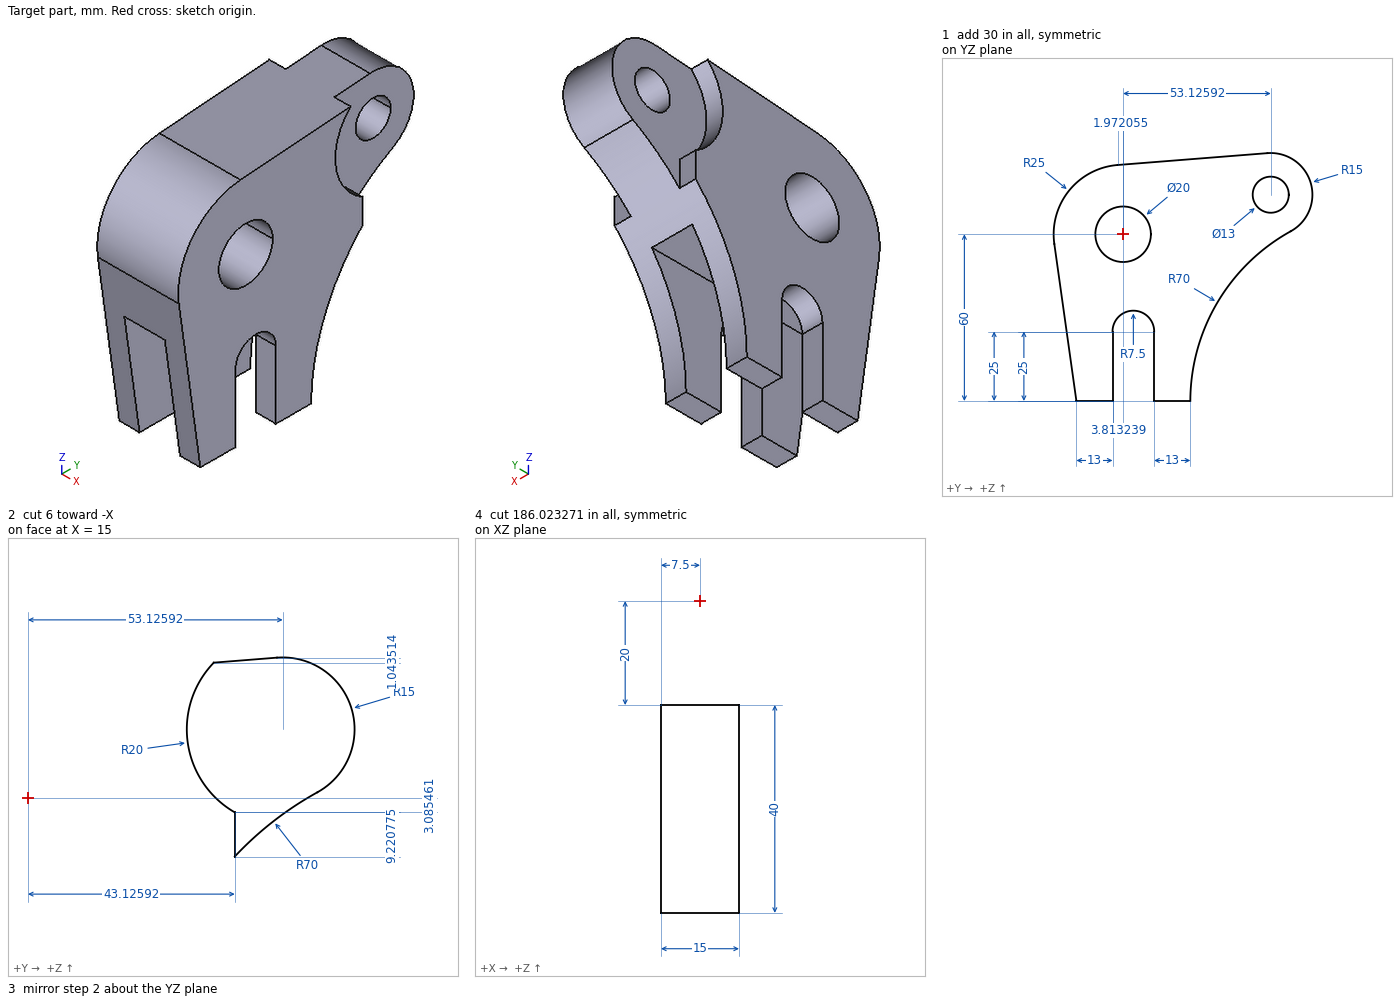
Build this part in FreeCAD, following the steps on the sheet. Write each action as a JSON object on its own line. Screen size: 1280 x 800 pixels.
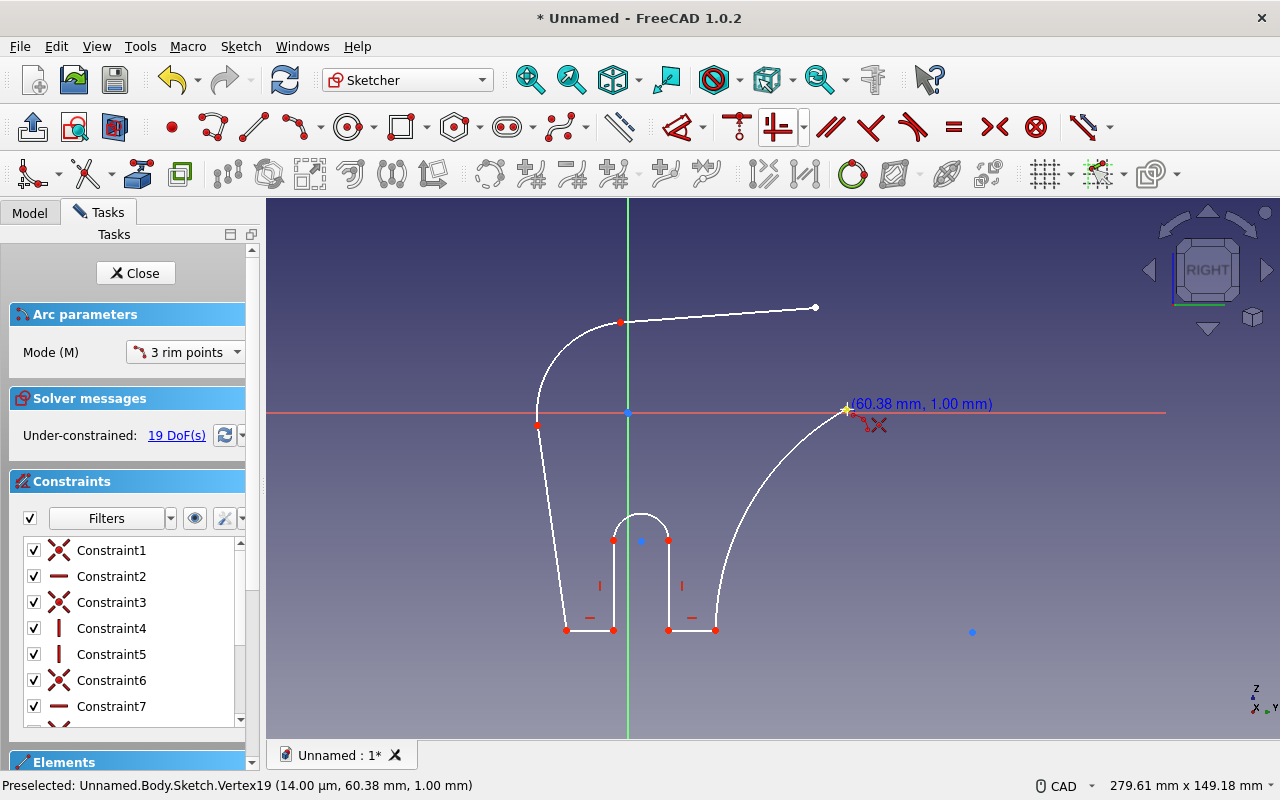
{"action": "left_click", "coordinate": [816, 308]}
{"action": "left_click", "coordinate": [872, 345]}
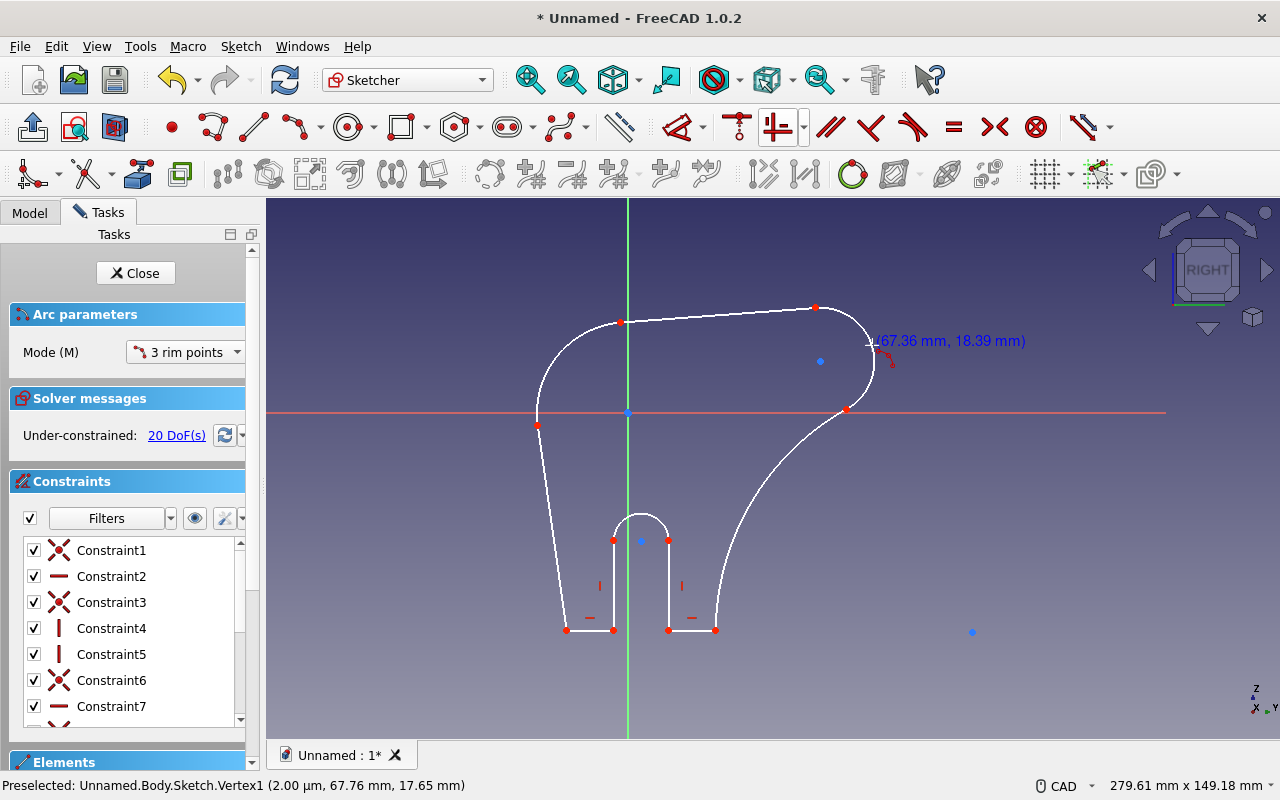
{"action": "left_click", "coordinate": [348, 128]}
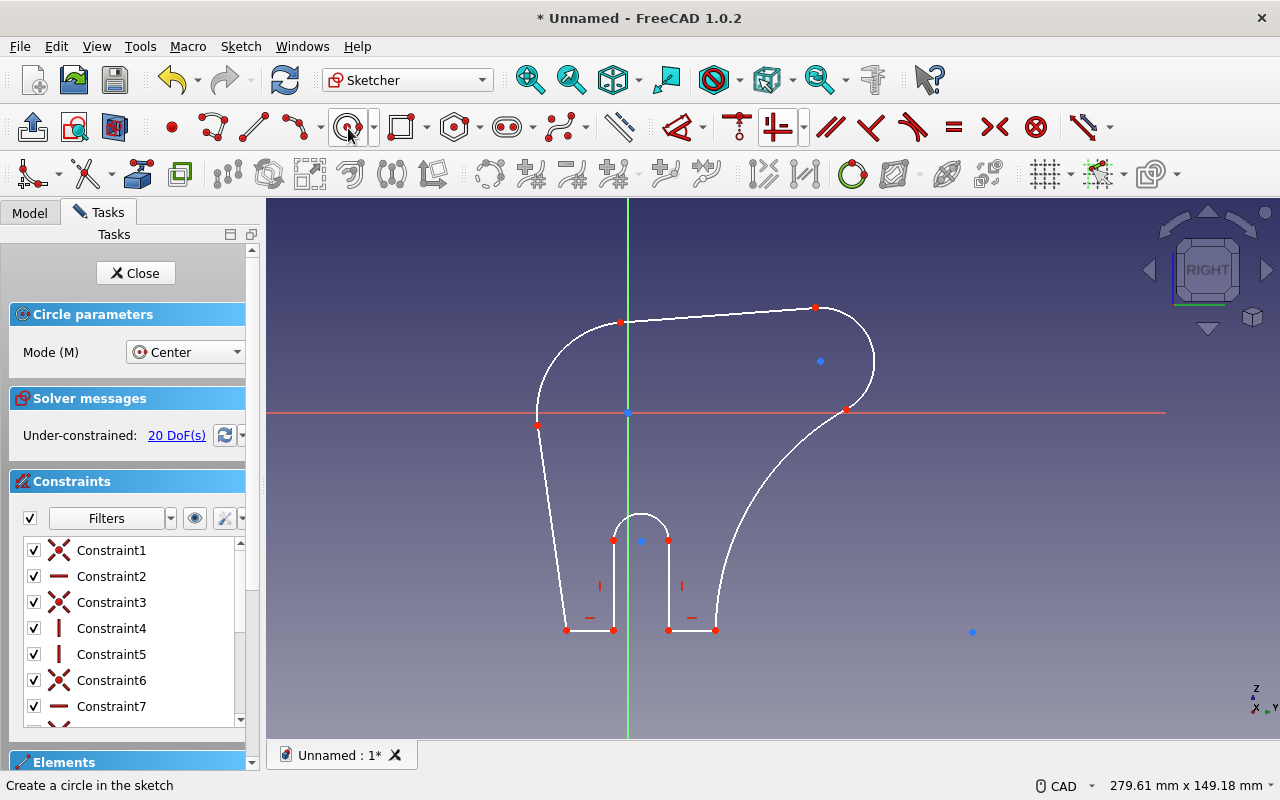
{"action": "left_click", "coordinate": [628, 413]}
{"action": "mouse_move", "coordinate": [653, 387]}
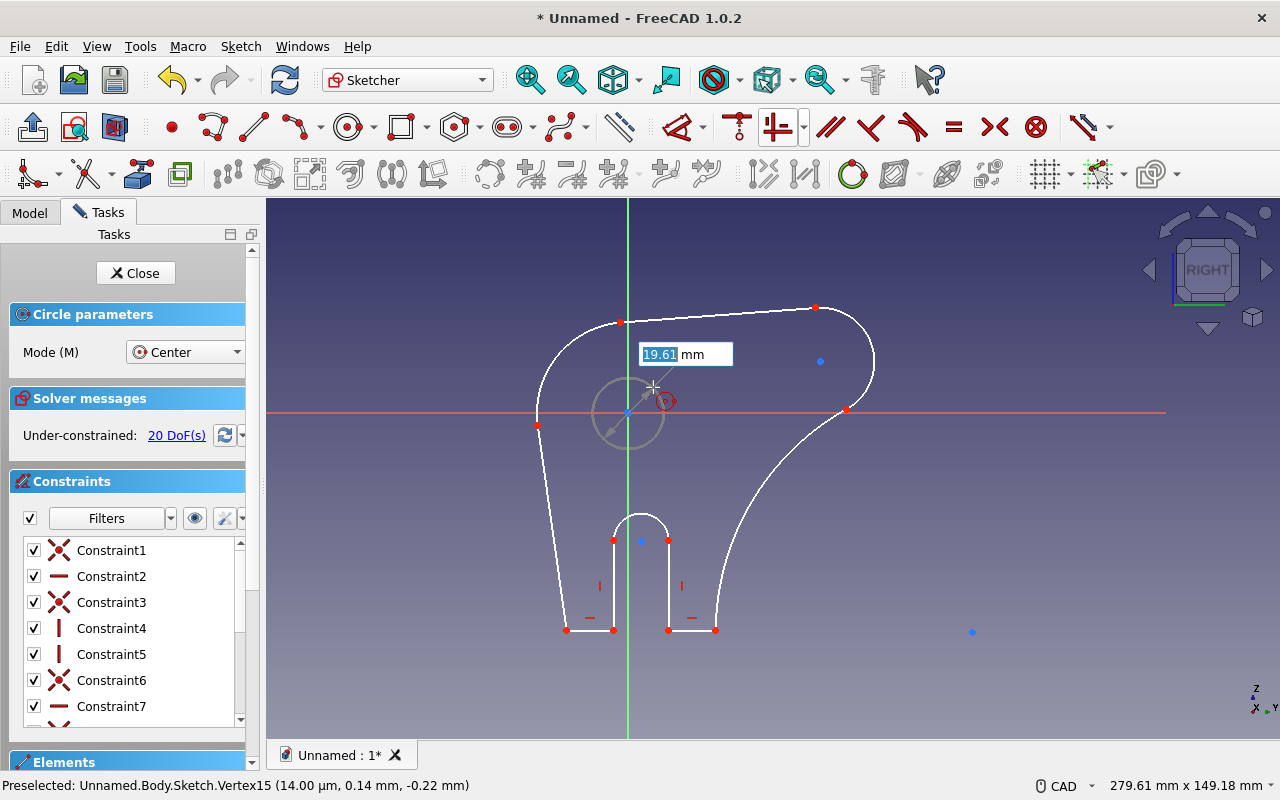
{"action": "type", "text": "20"}
{"action": "key", "text": "Return"}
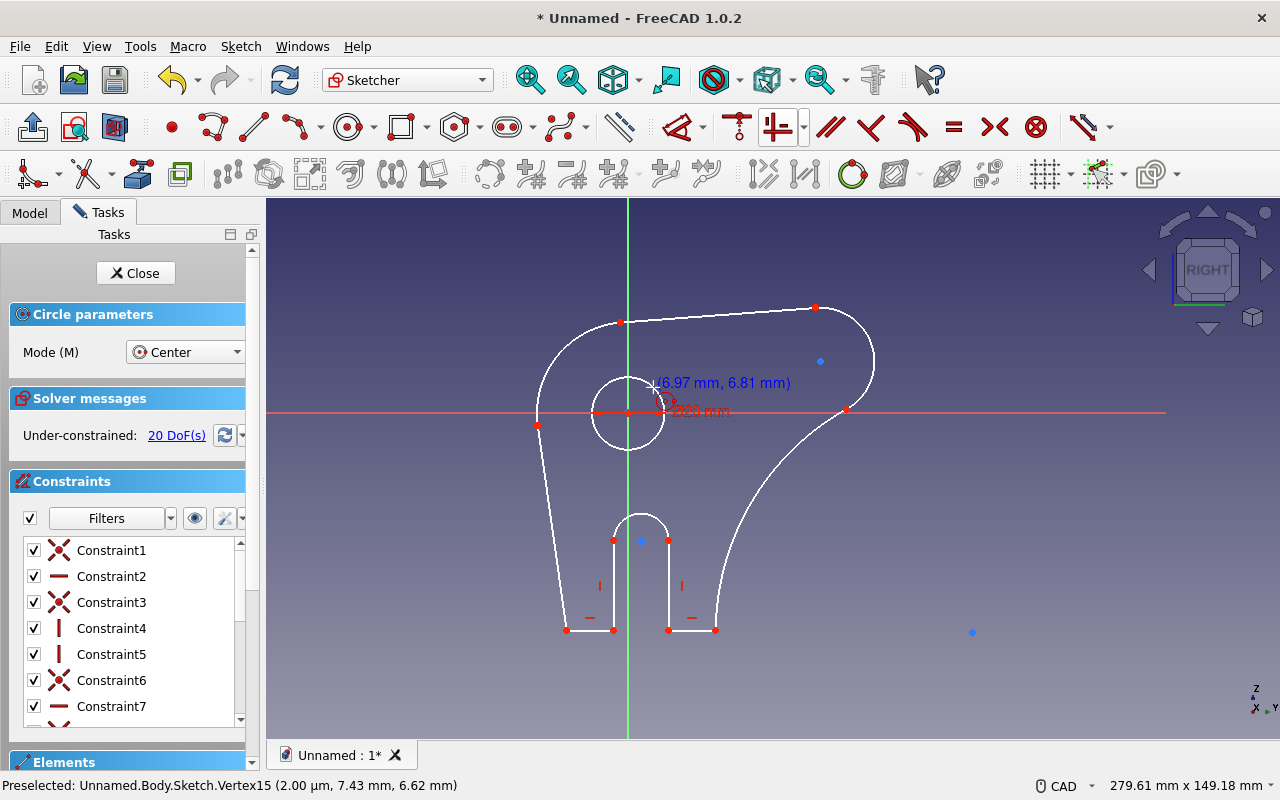
{"action": "left_click", "coordinate": [820, 361]}
{"action": "mouse_move", "coordinate": [837, 344]}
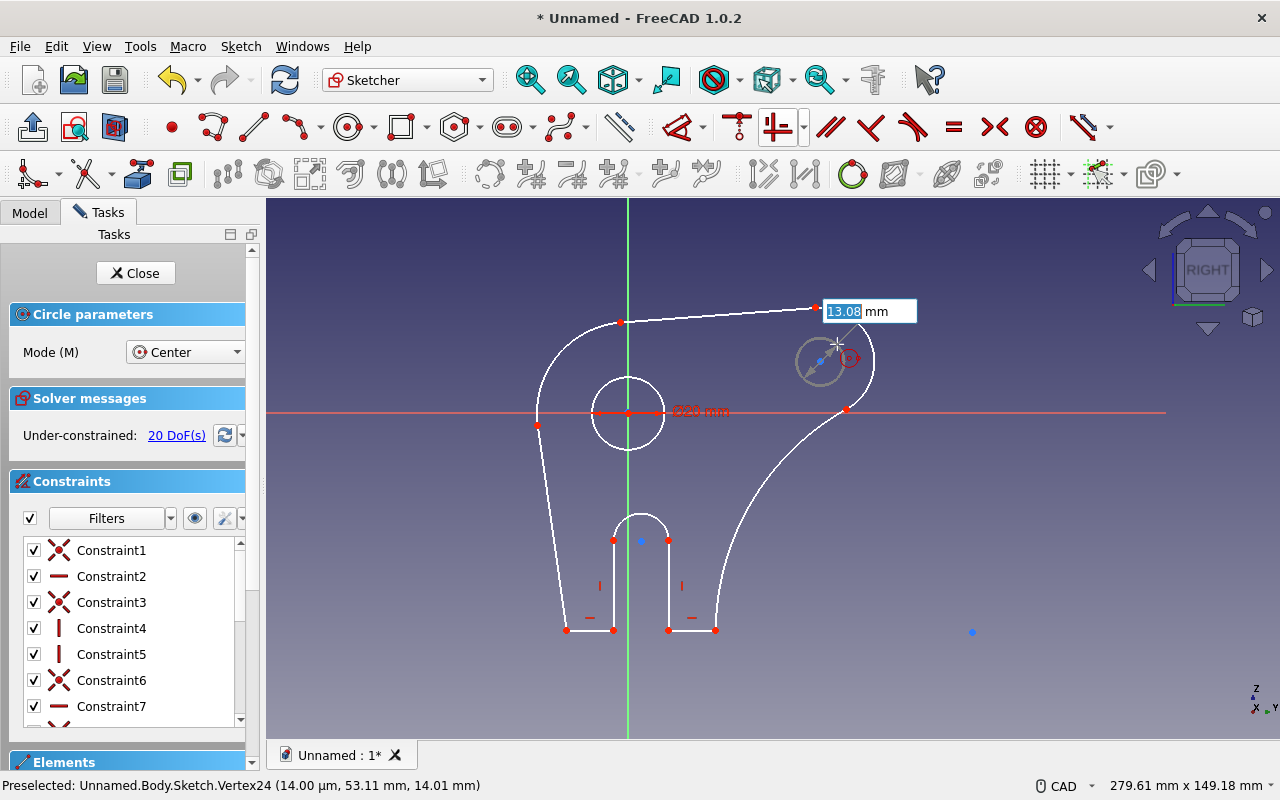
{"action": "type", "text": "13"}
{"action": "key", "text": "Return"}
{"action": "key", "text": "Escape"}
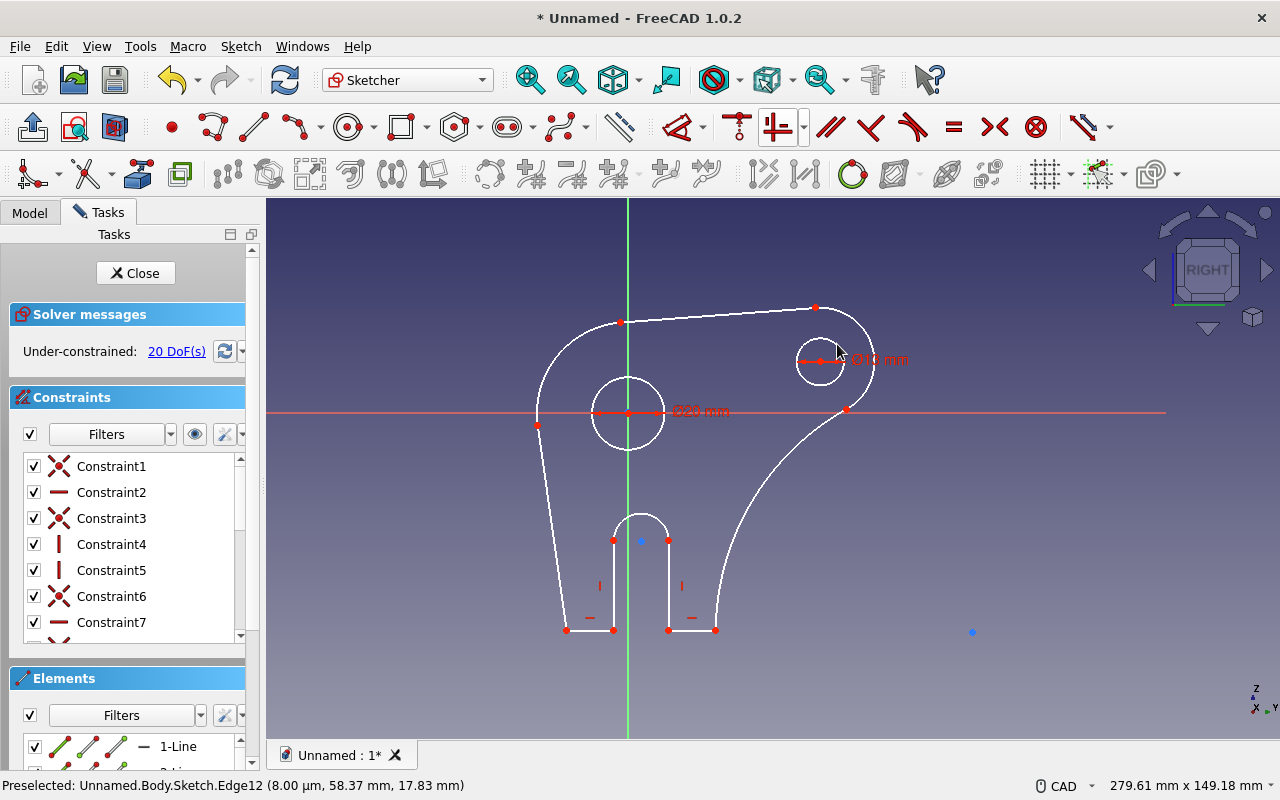
{"action": "left_click", "coordinate": [757, 312]}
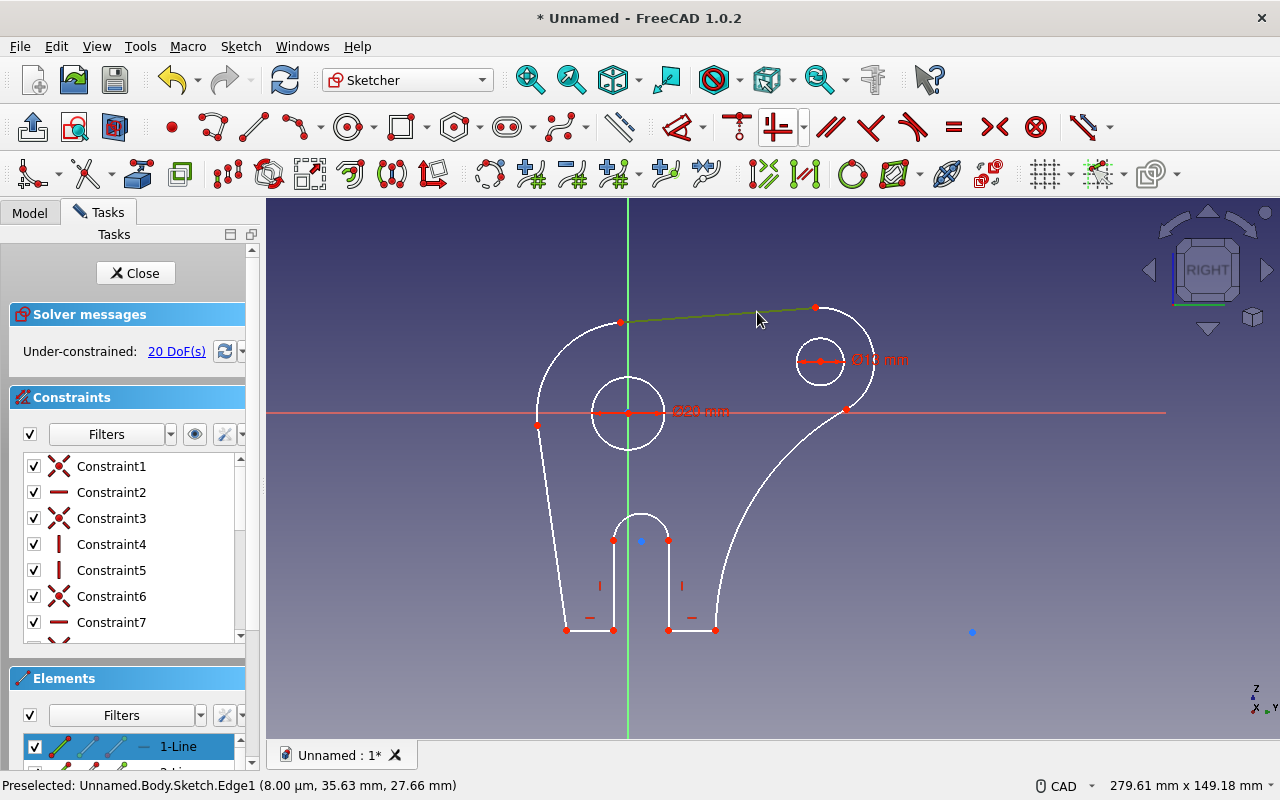
{"action": "left_click", "coordinate": [579, 337]}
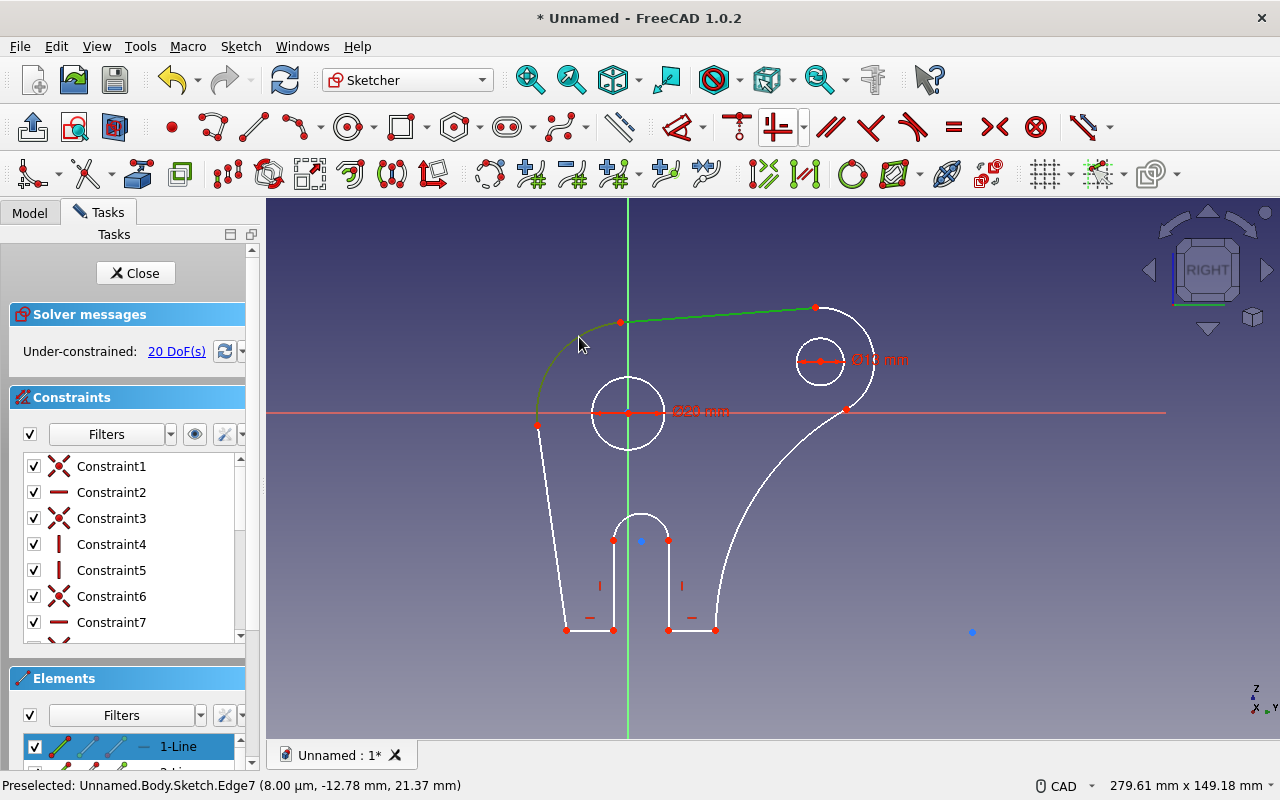
{"action": "left_click", "coordinate": [913, 128]}